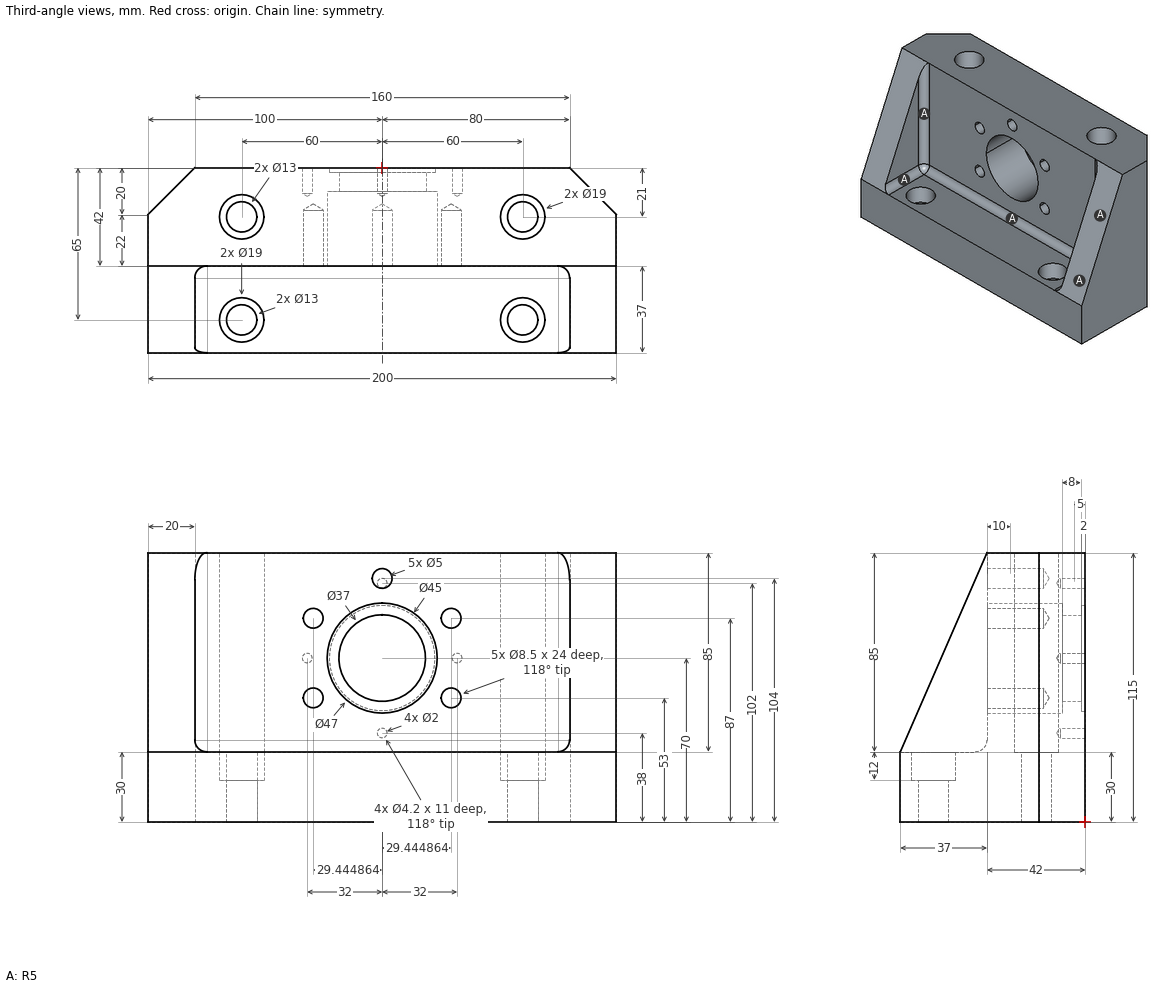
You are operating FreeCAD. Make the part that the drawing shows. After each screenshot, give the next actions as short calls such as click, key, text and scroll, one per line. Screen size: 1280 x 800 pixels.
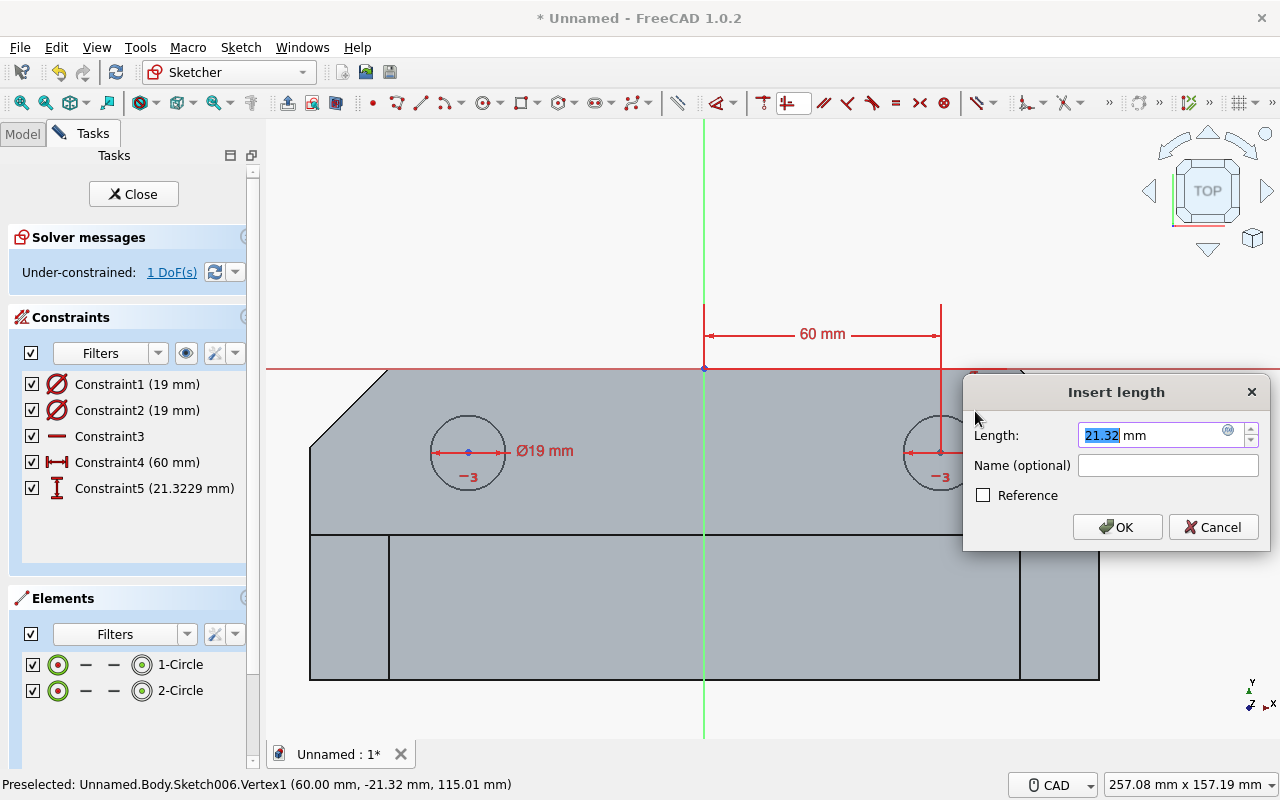
text(21)
key(Return)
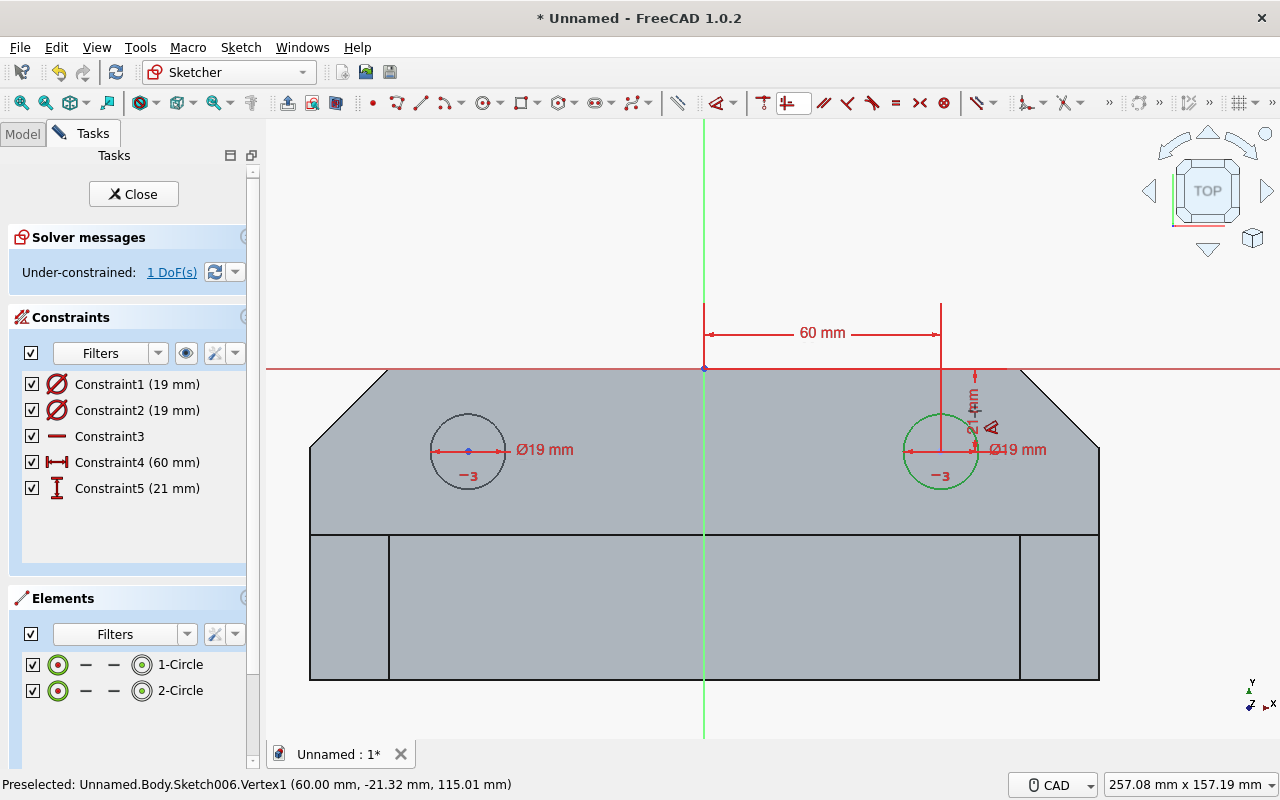
click(468, 452)
click(586, 335)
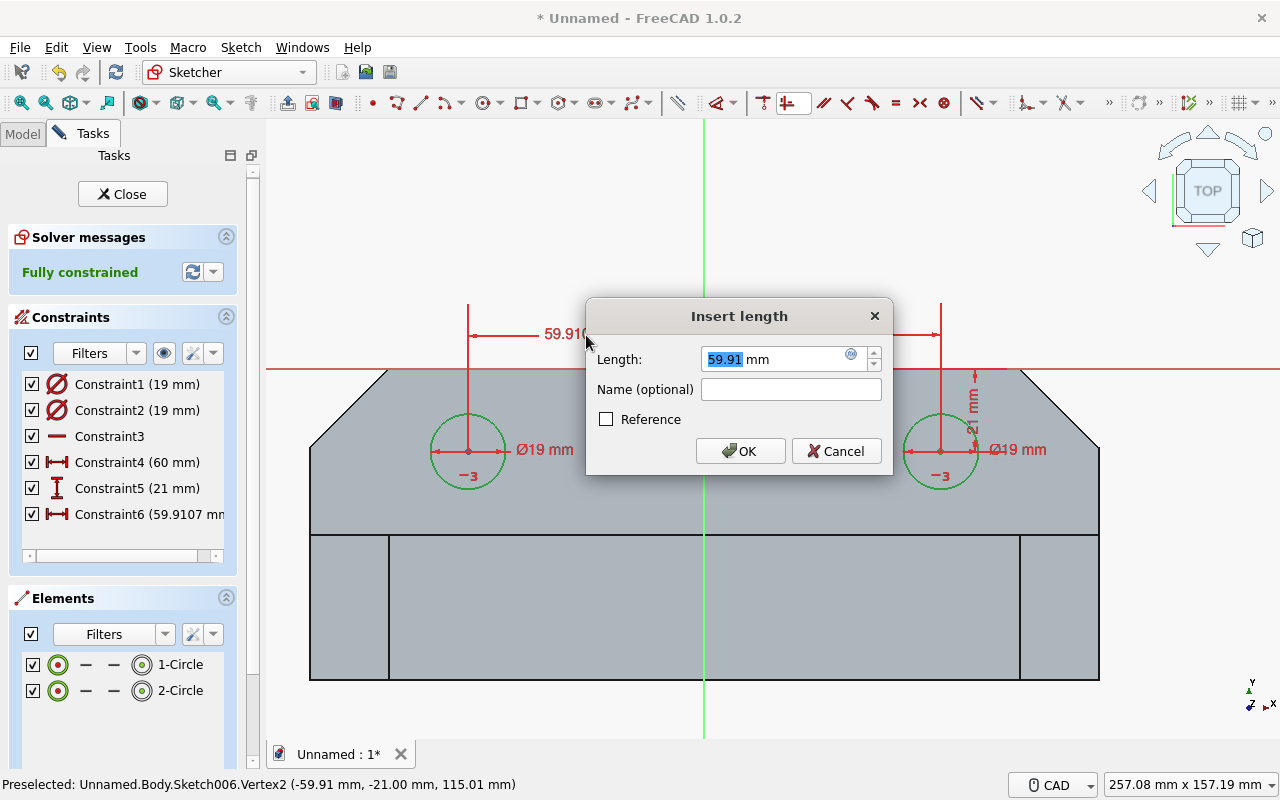
text(60)
key(Return)
key(Escape)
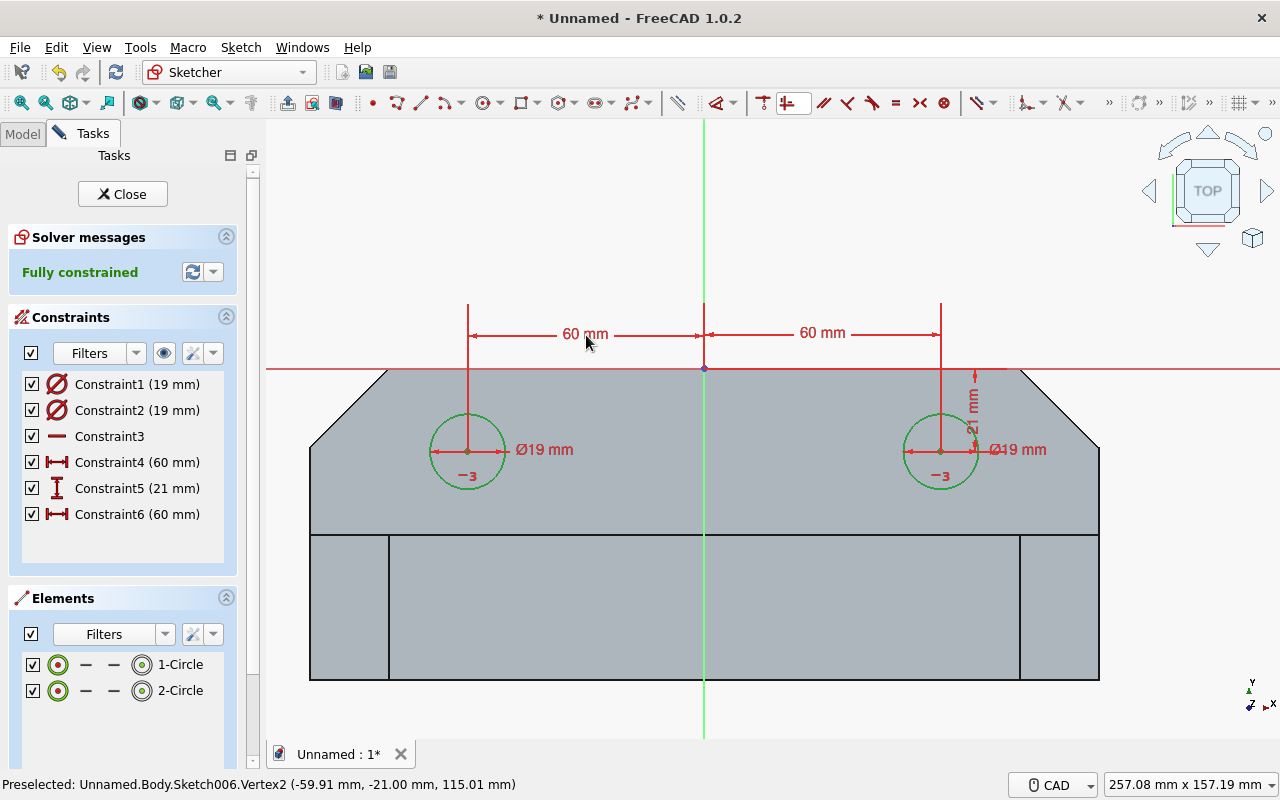
click(123, 194)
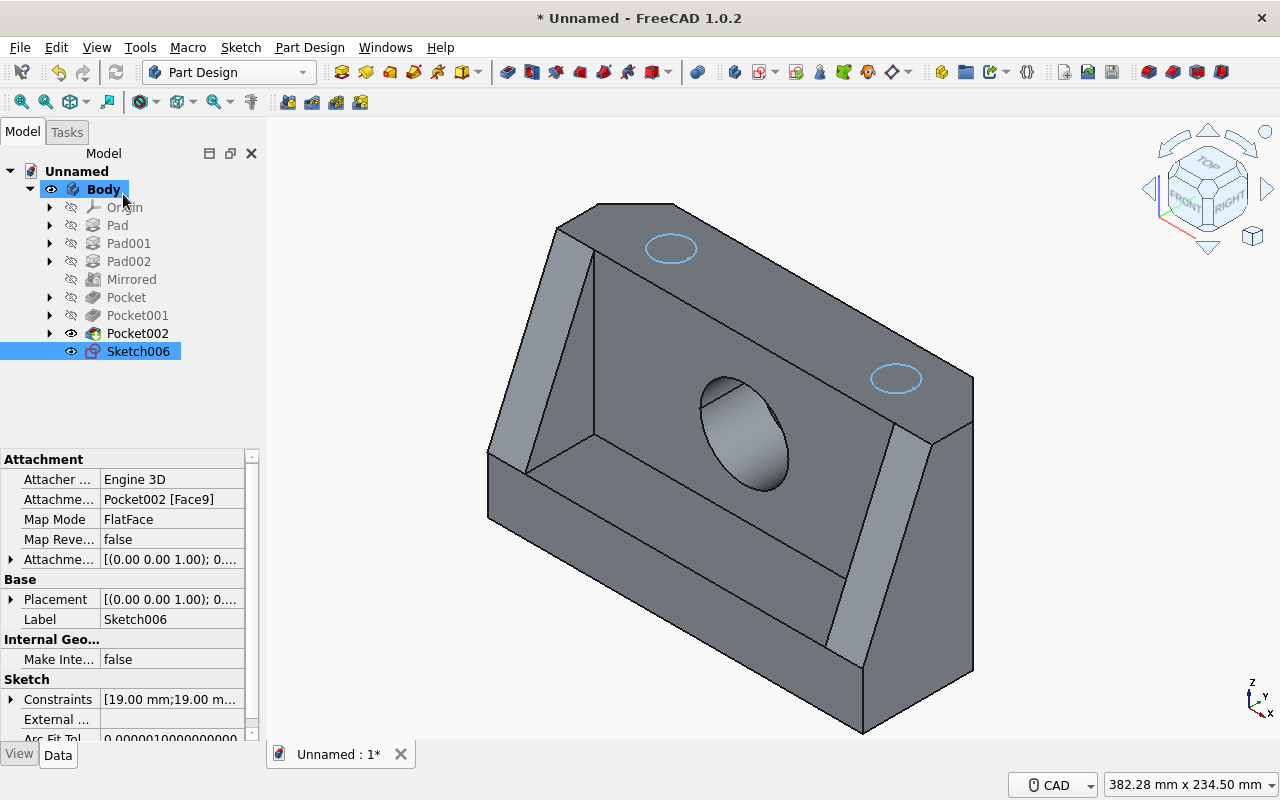
click(508, 72)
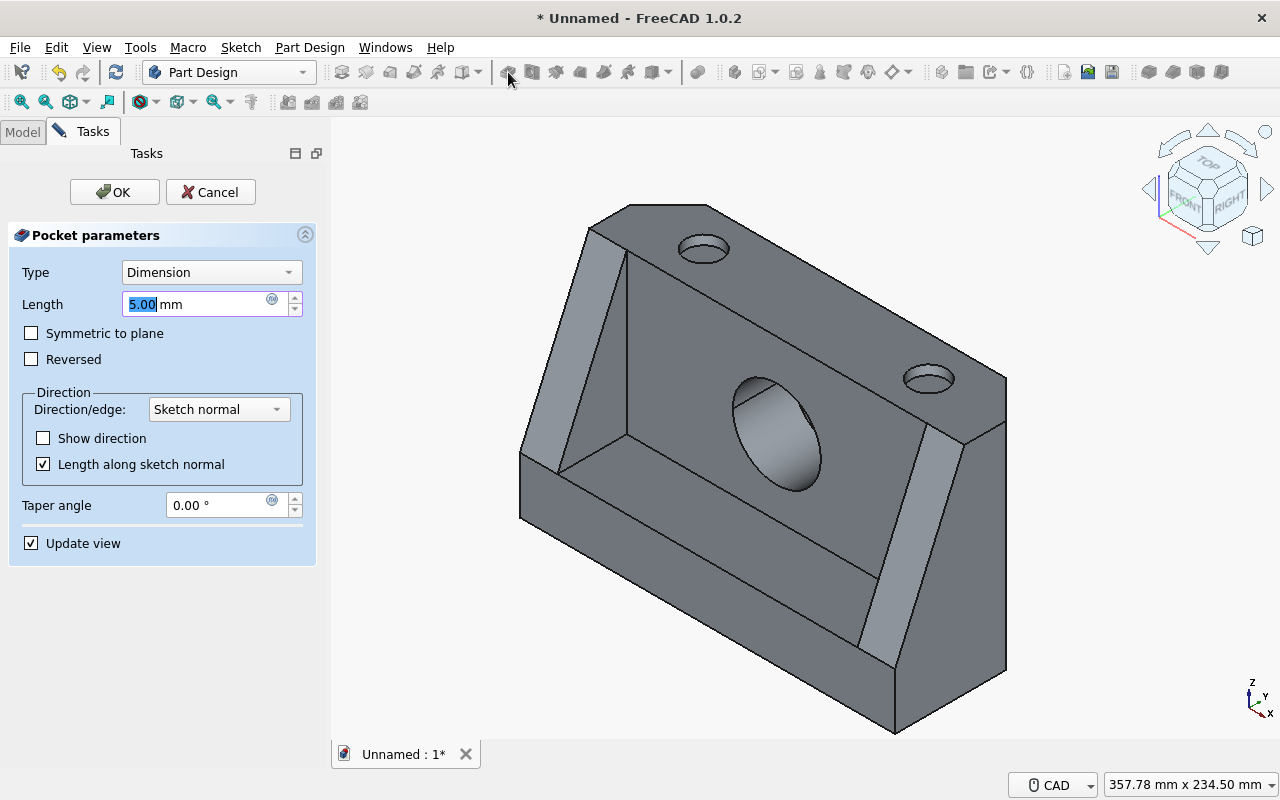
text(85)
key(Tab)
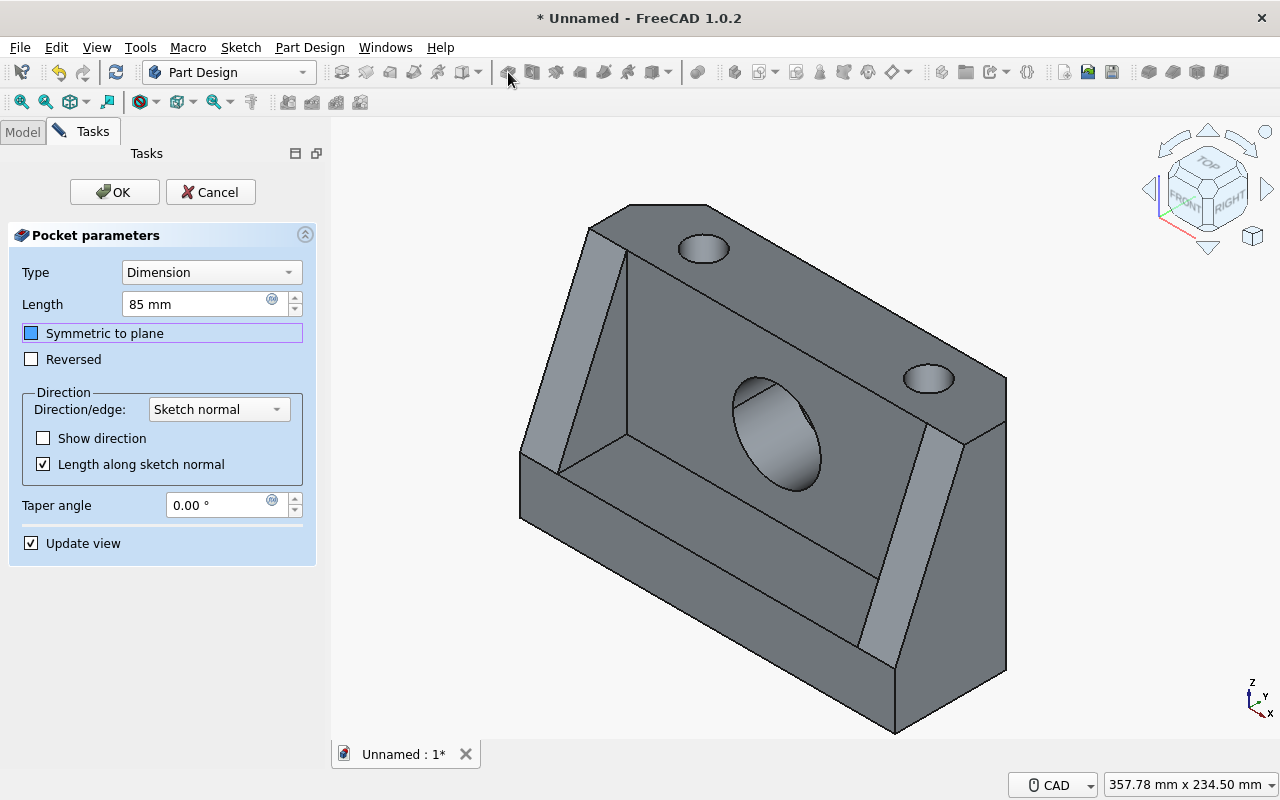
click(115, 192)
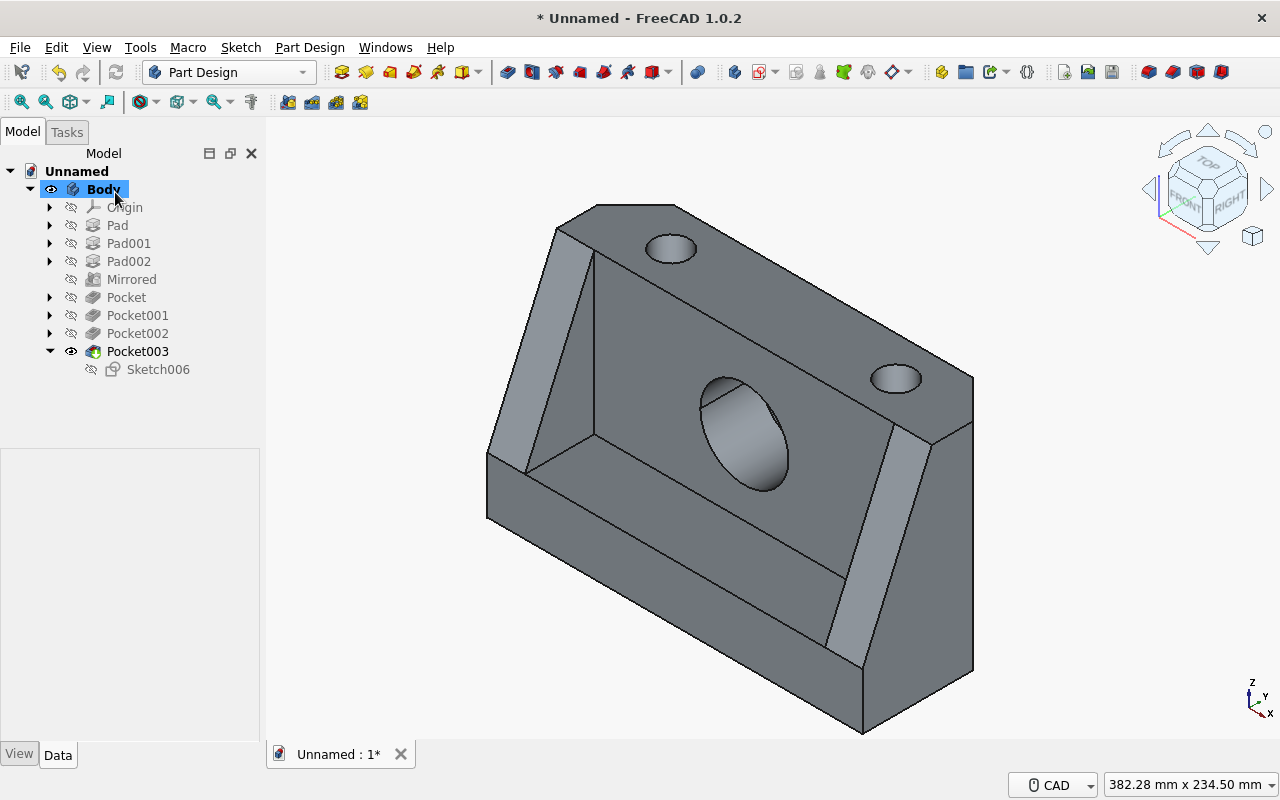
click(795, 589)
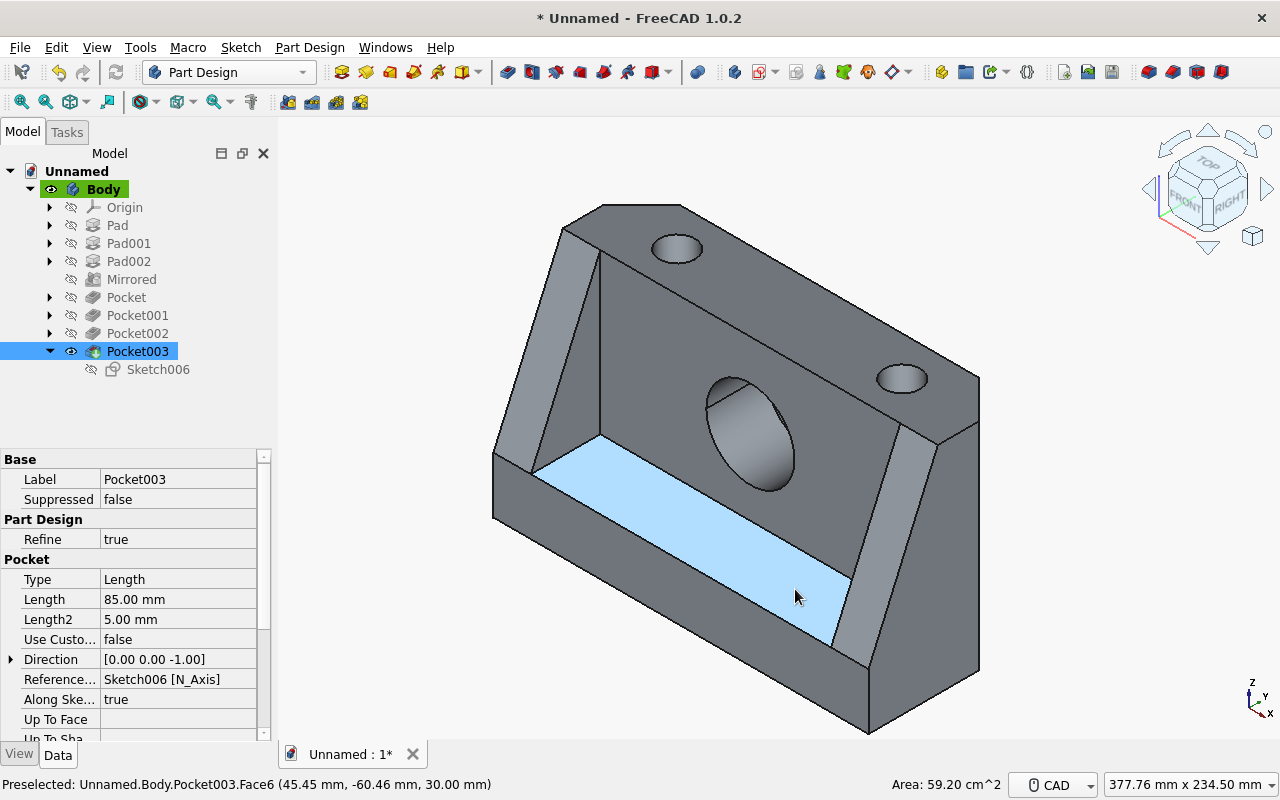
click(760, 72)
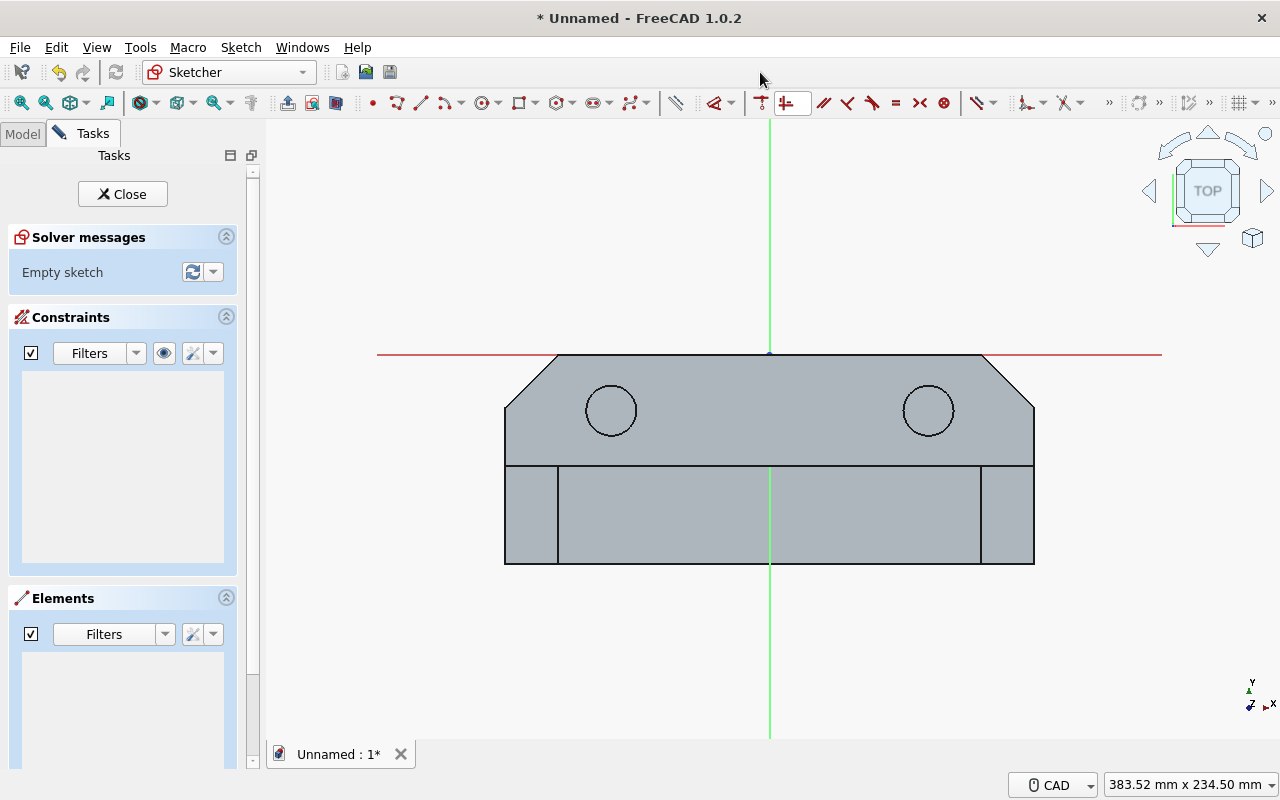
click(336, 104)